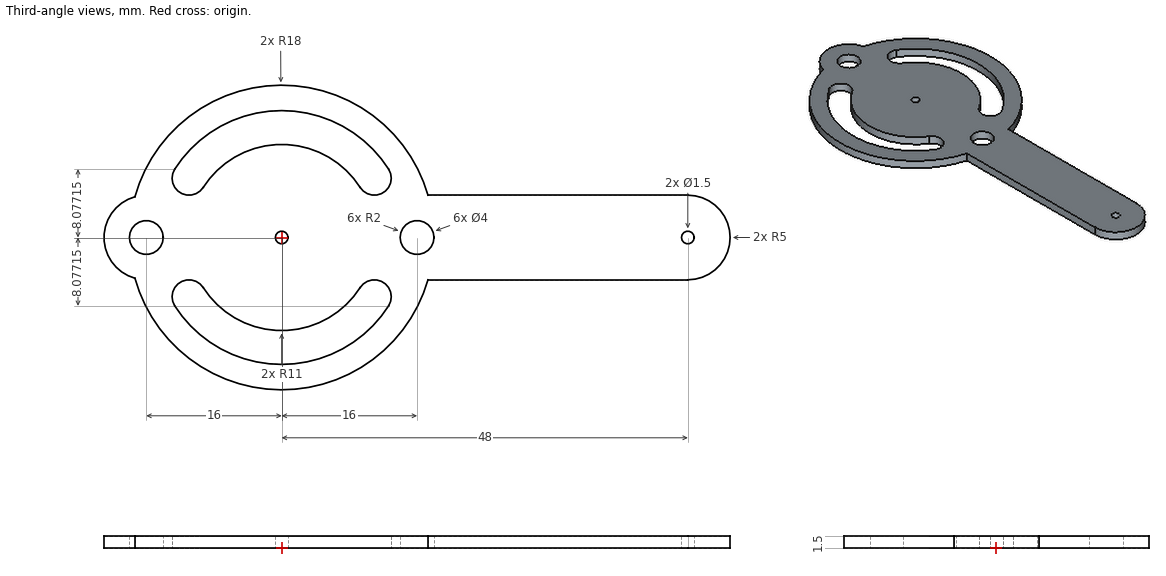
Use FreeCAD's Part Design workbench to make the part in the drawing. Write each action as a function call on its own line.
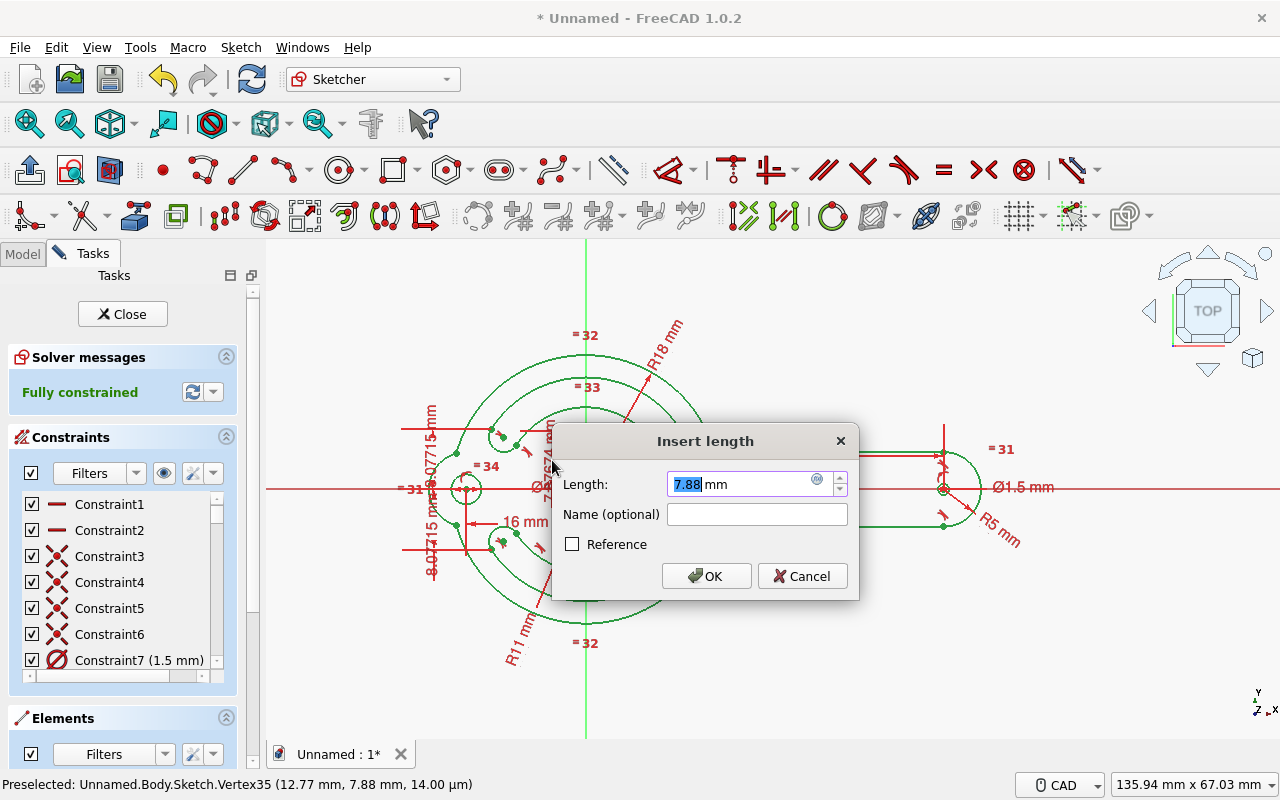
text(8.07715)
key(Return)
key(Escape)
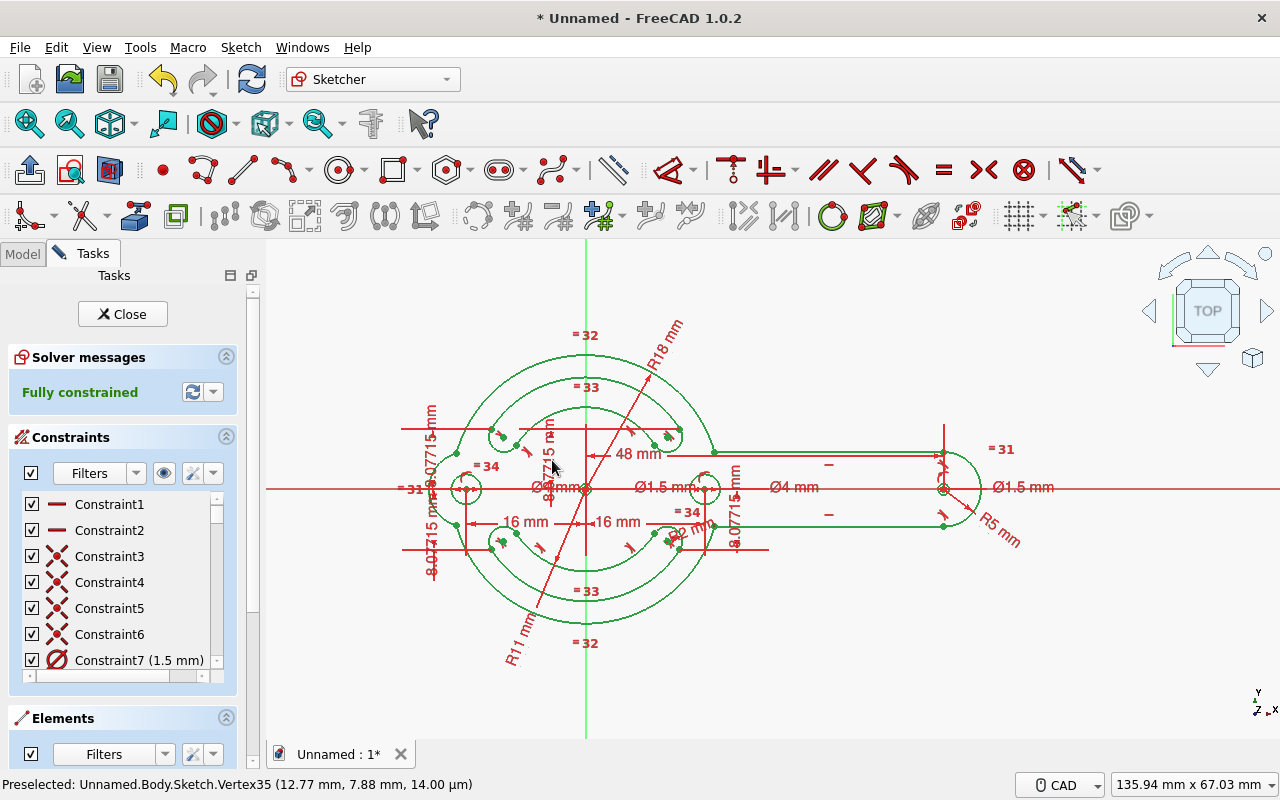
click(123, 314)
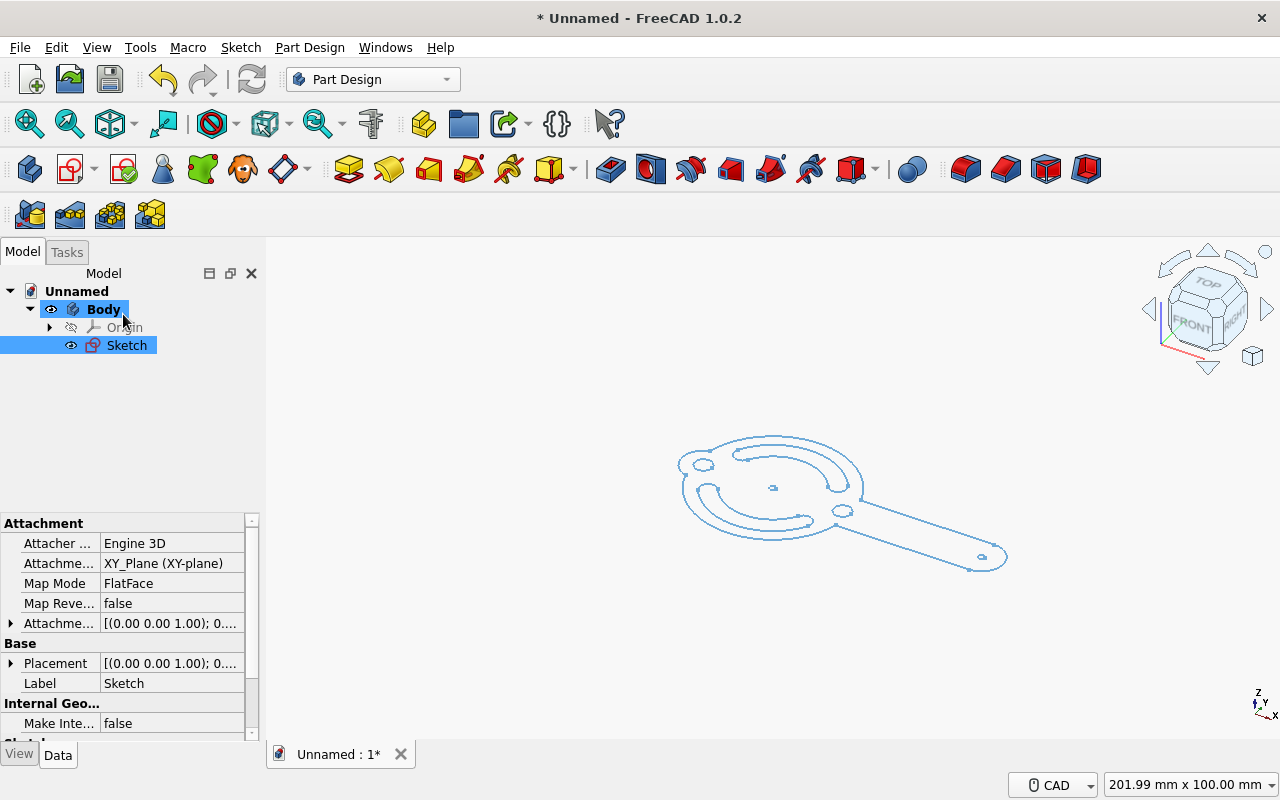
click(350, 170)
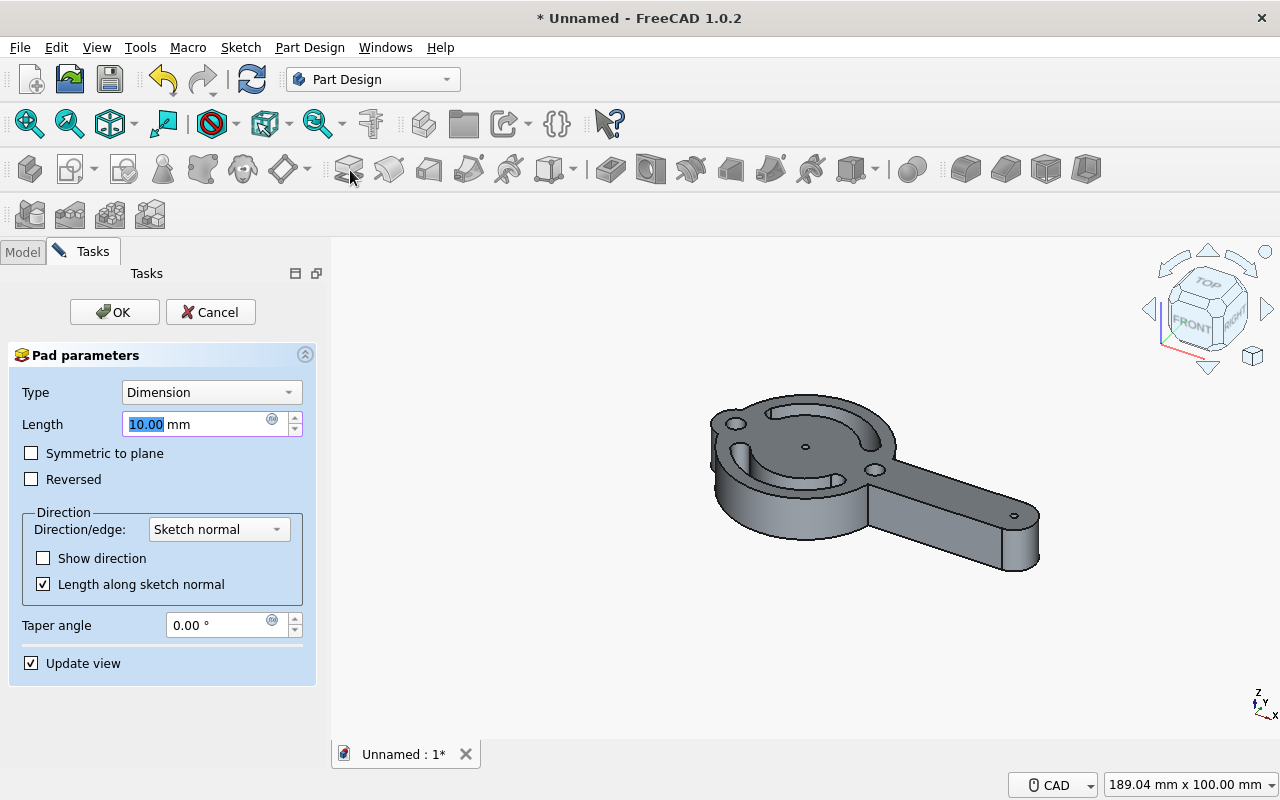
text(1.5)
key(Tab)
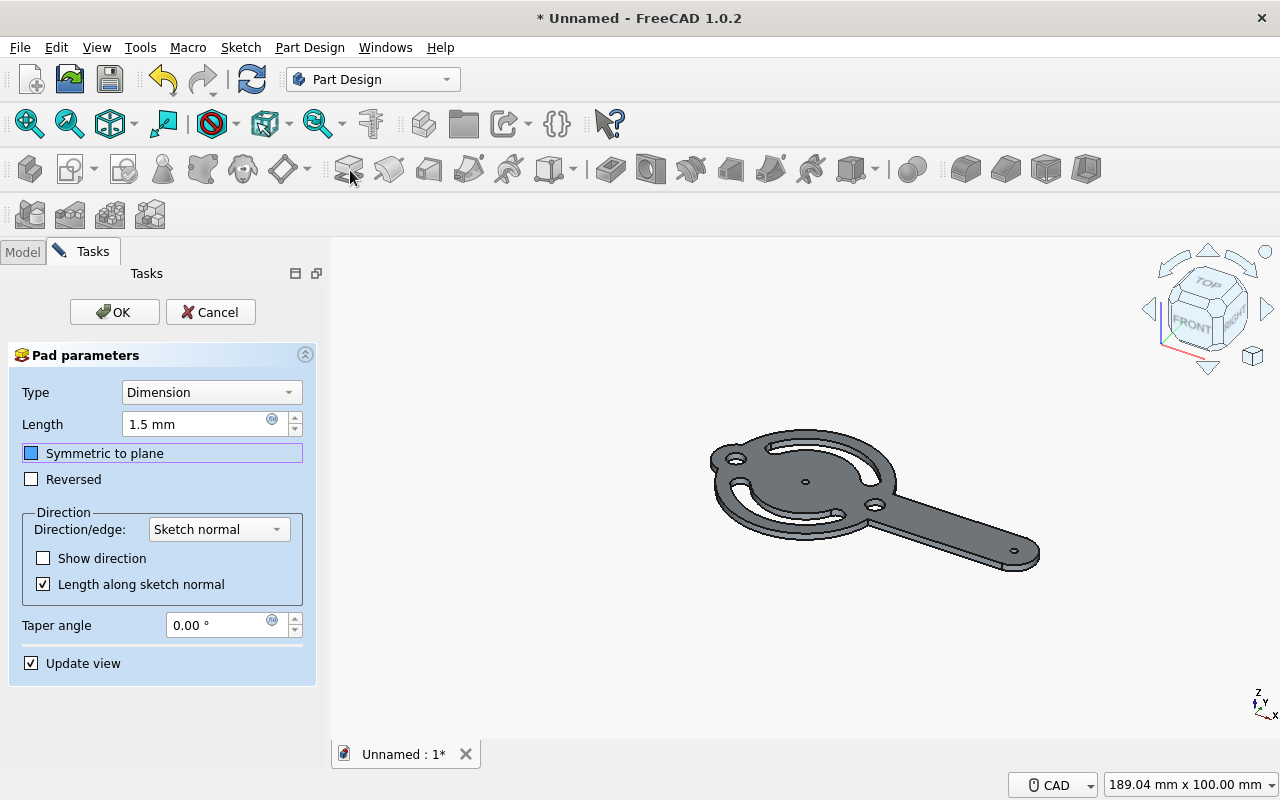
click(115, 312)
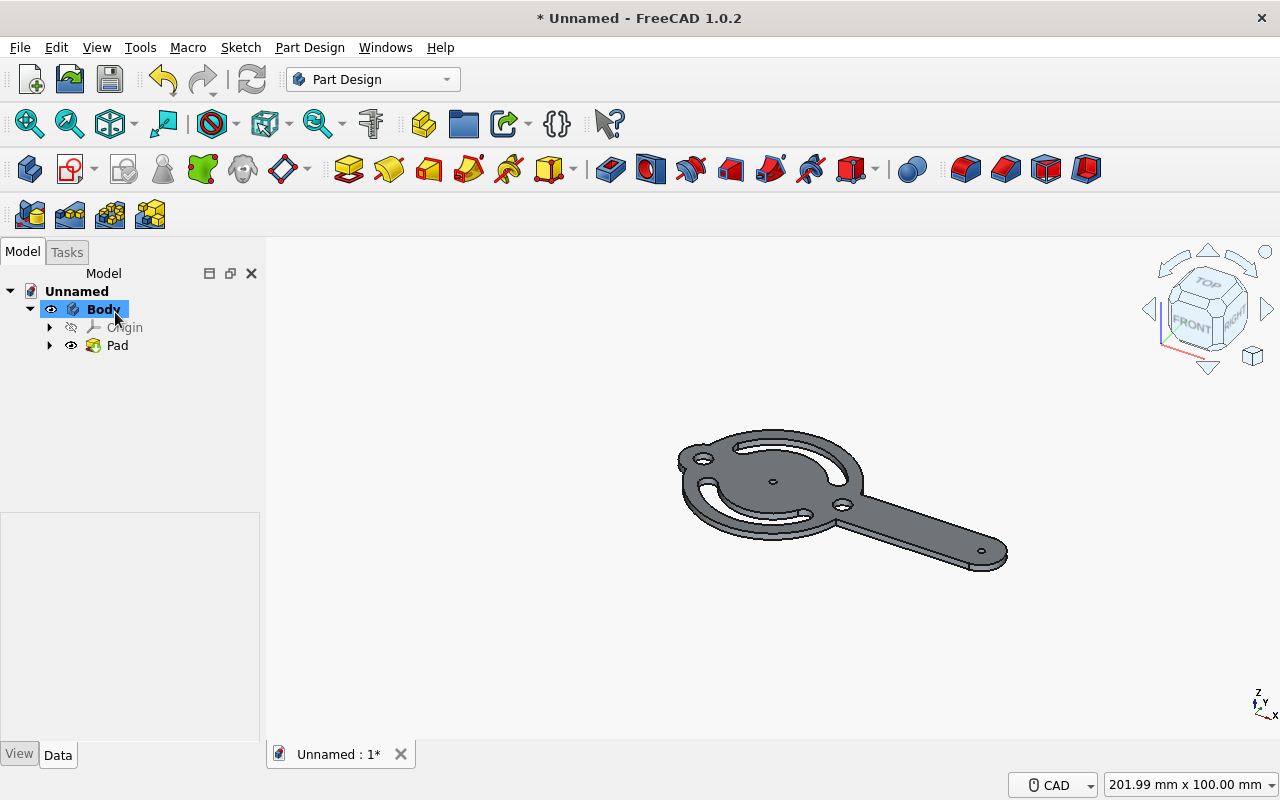
key(0)